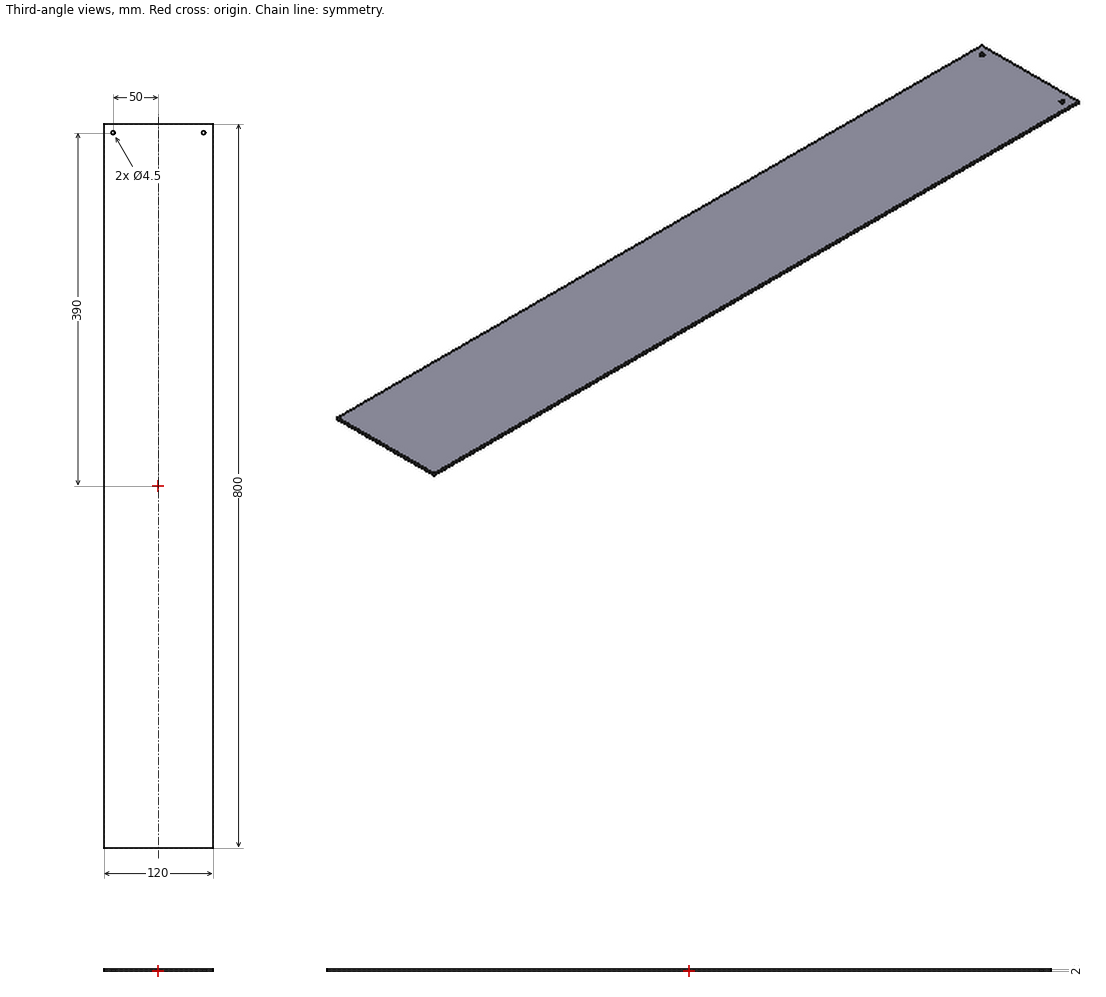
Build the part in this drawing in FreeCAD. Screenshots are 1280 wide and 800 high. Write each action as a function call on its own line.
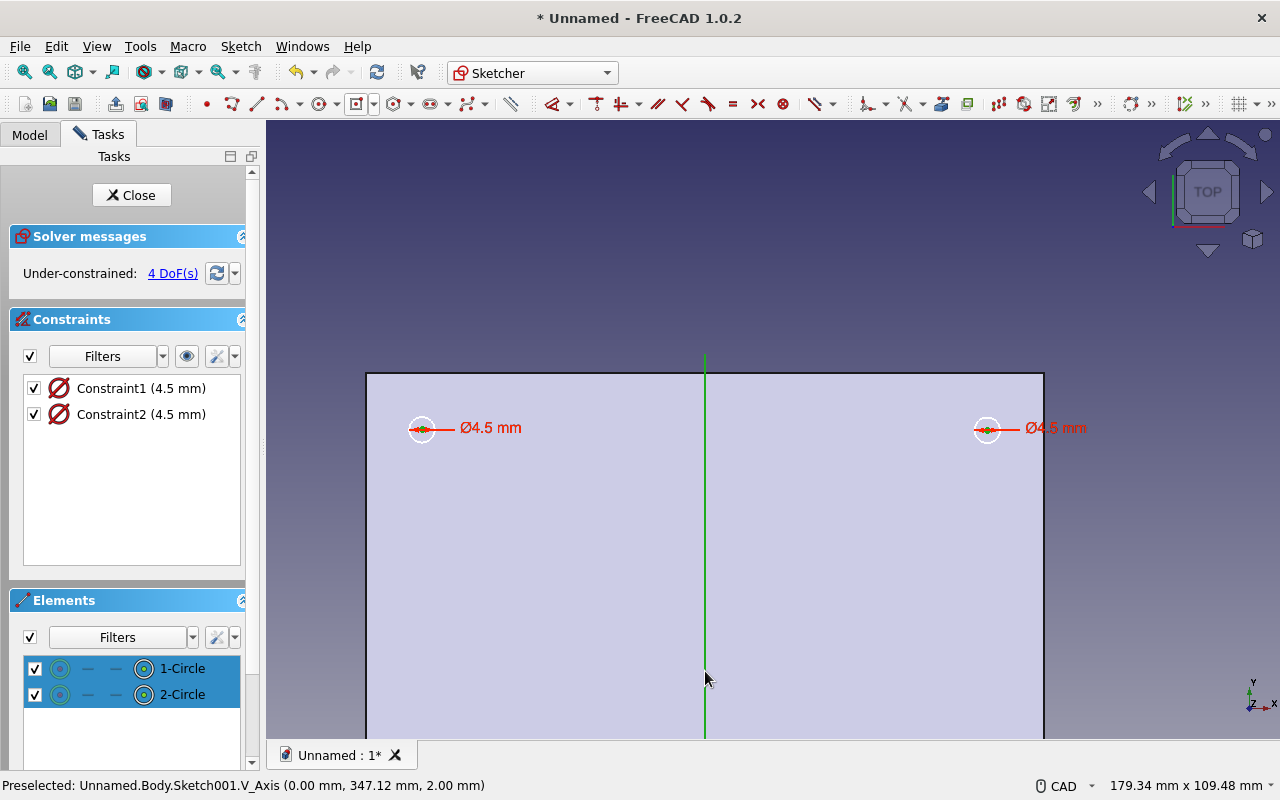
key(s)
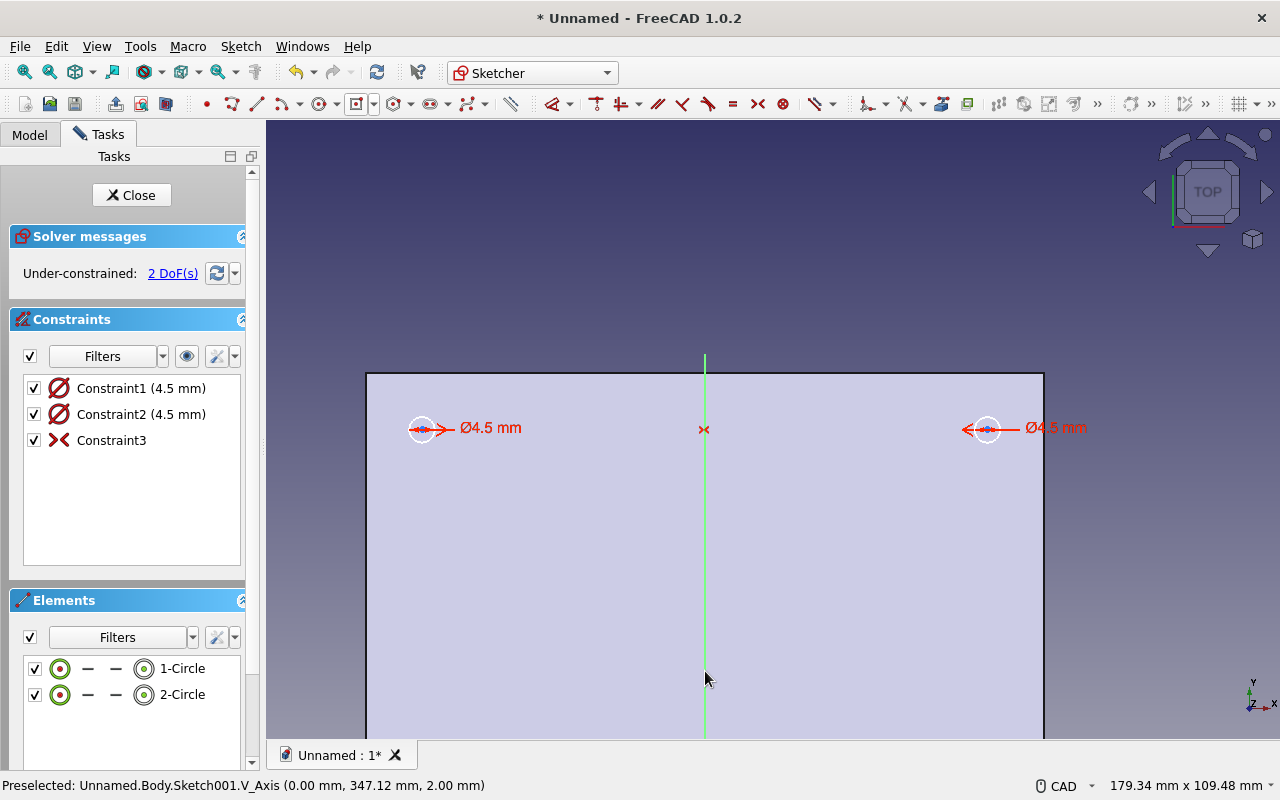
click(552, 104)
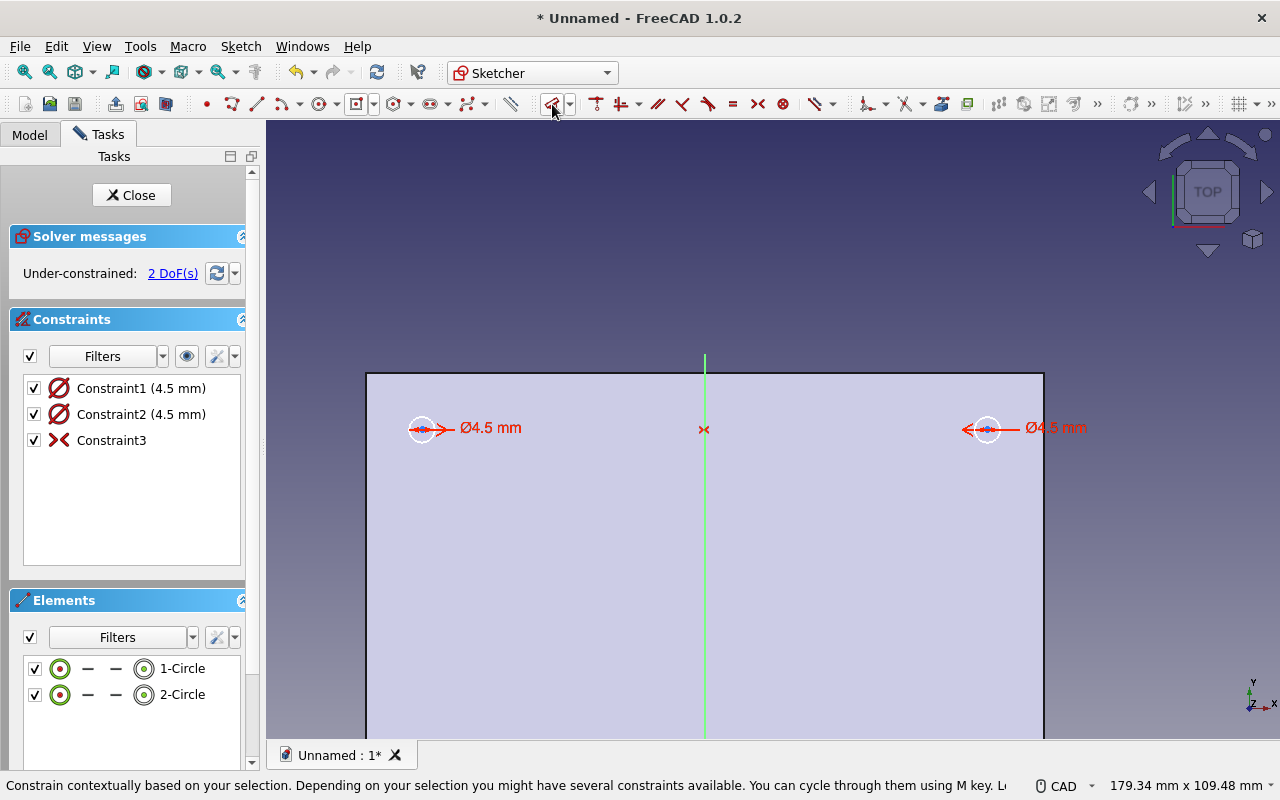
click(422, 430)
click(563, 396)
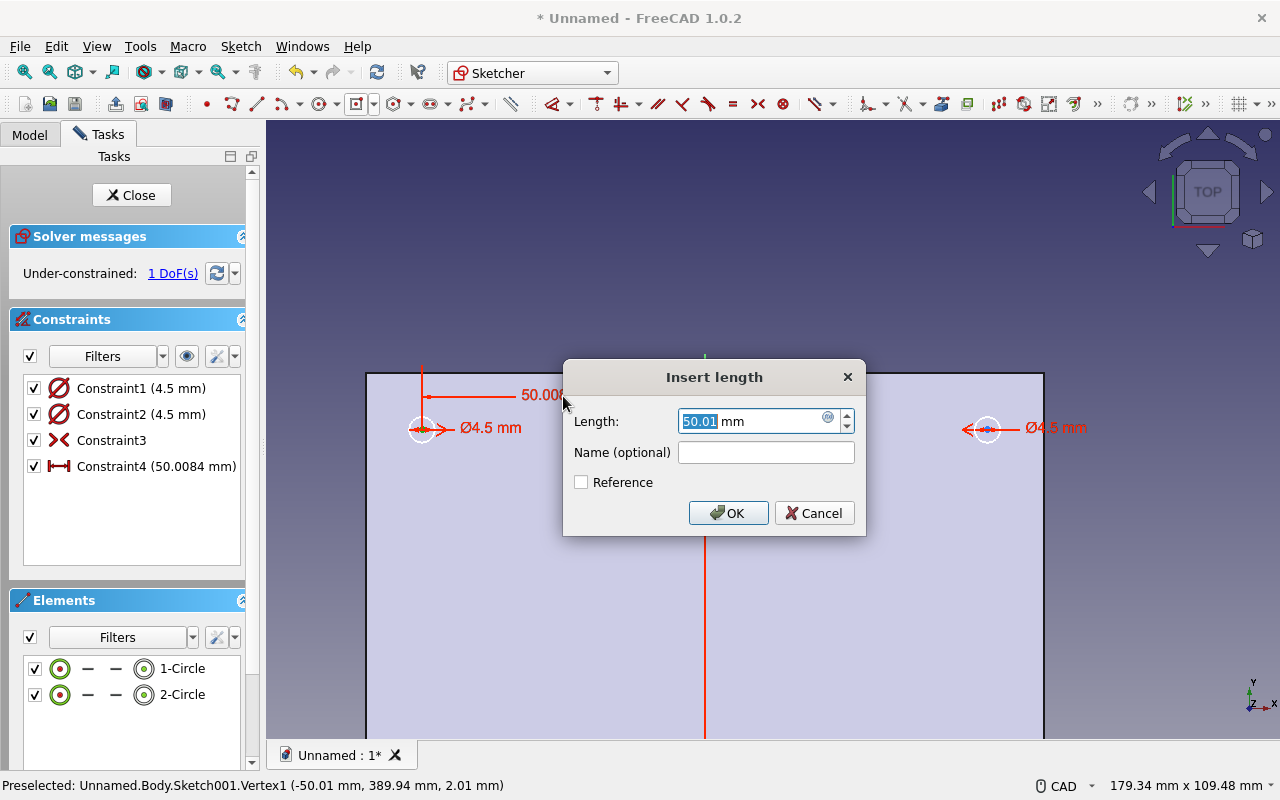
text(50)
key(Return)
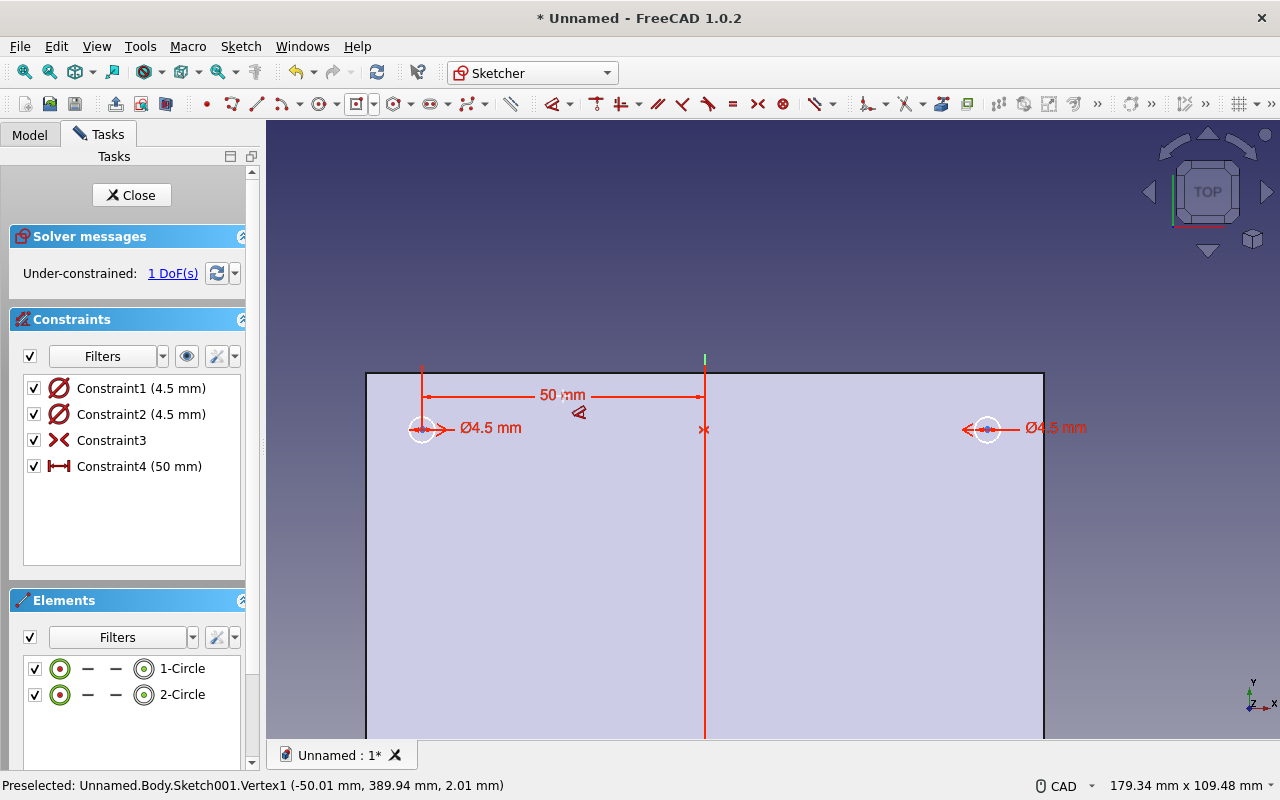
click(422, 430)
click(388, 570)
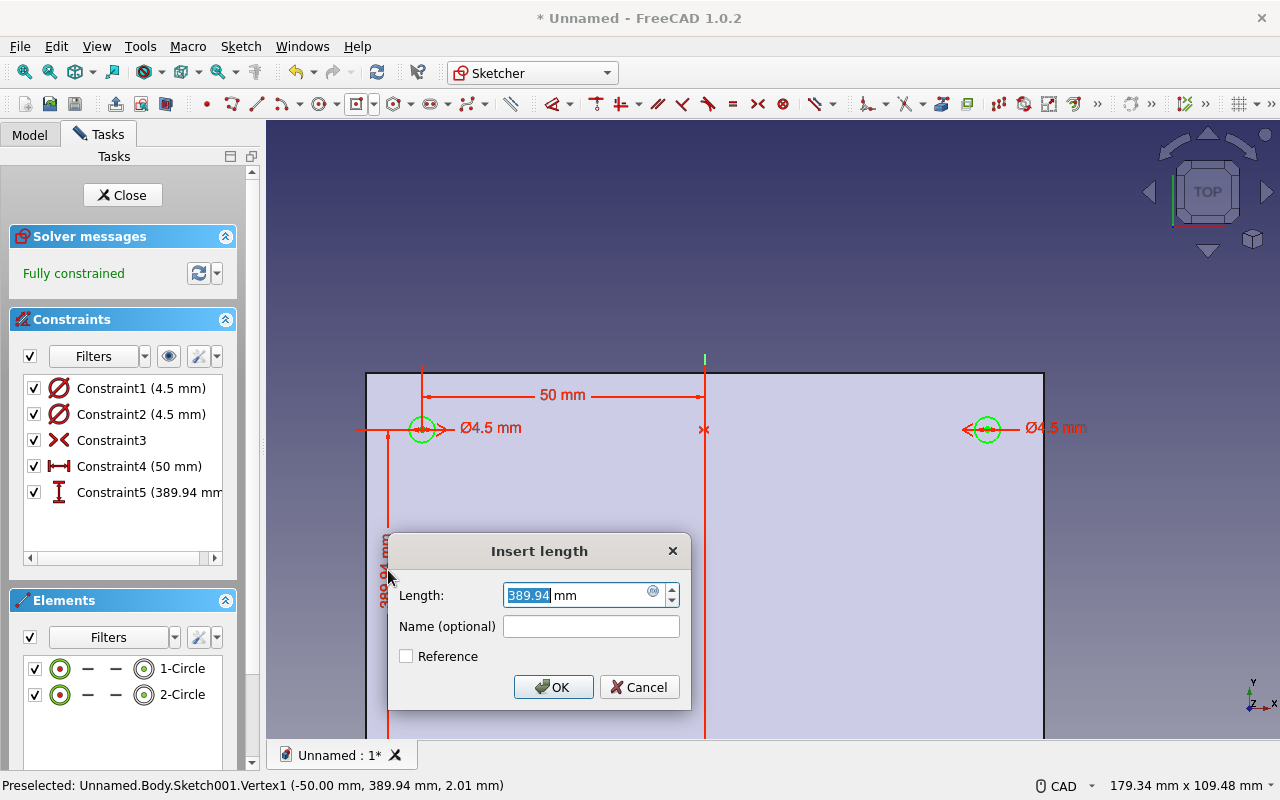
text(390)
key(Return)
key(Escape)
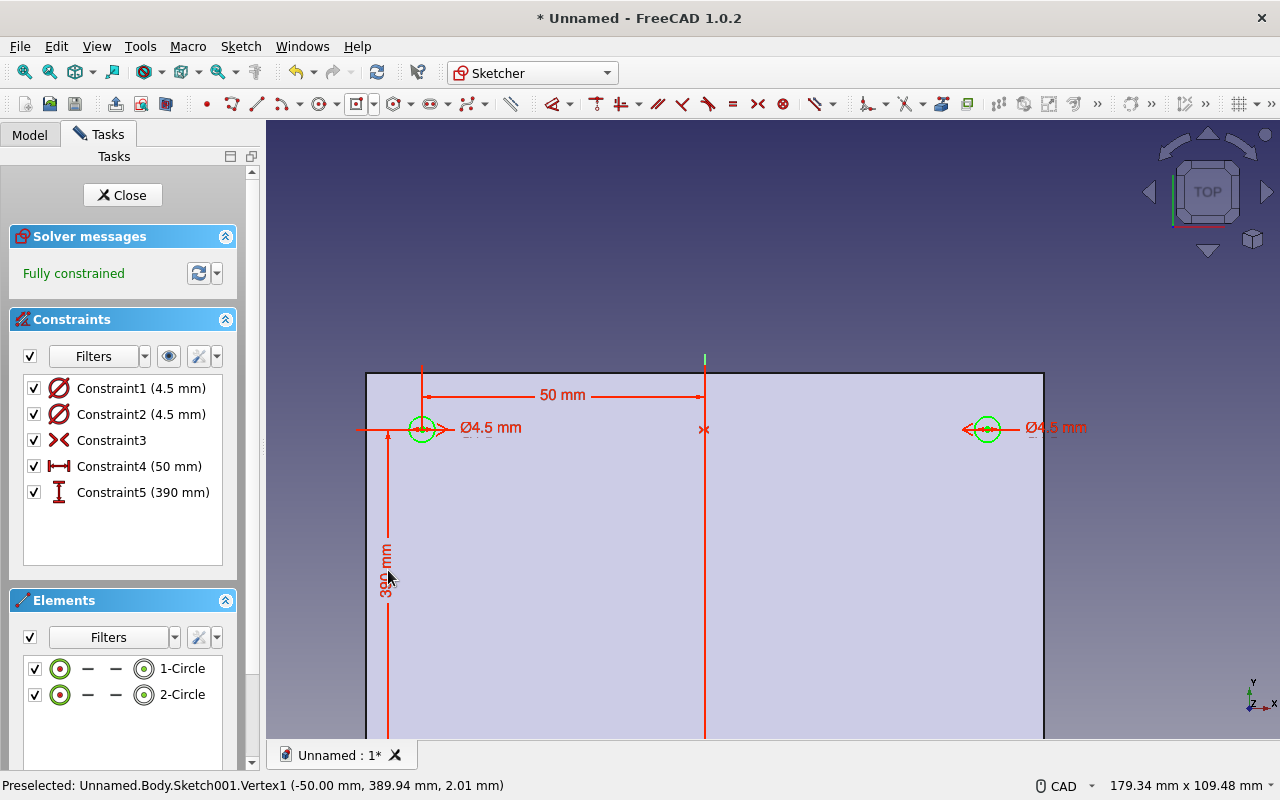
click(123, 195)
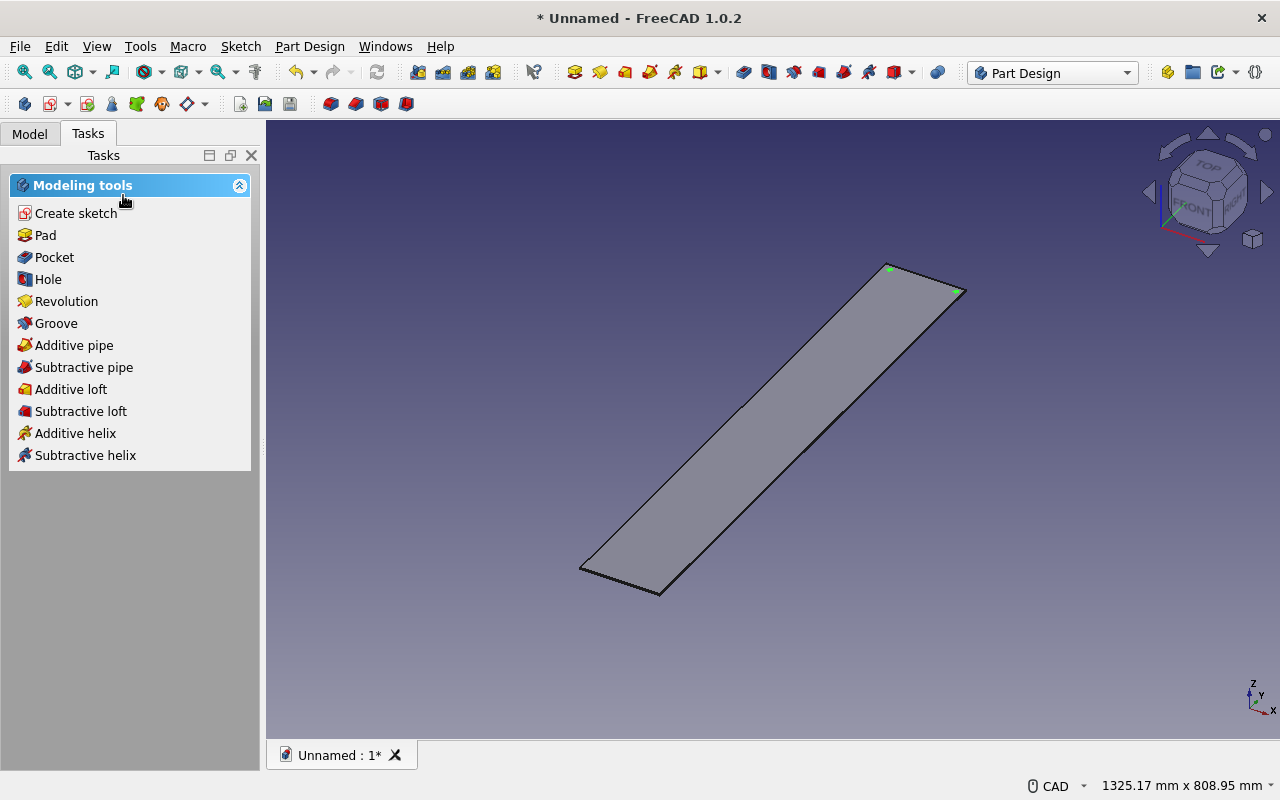
click(744, 72)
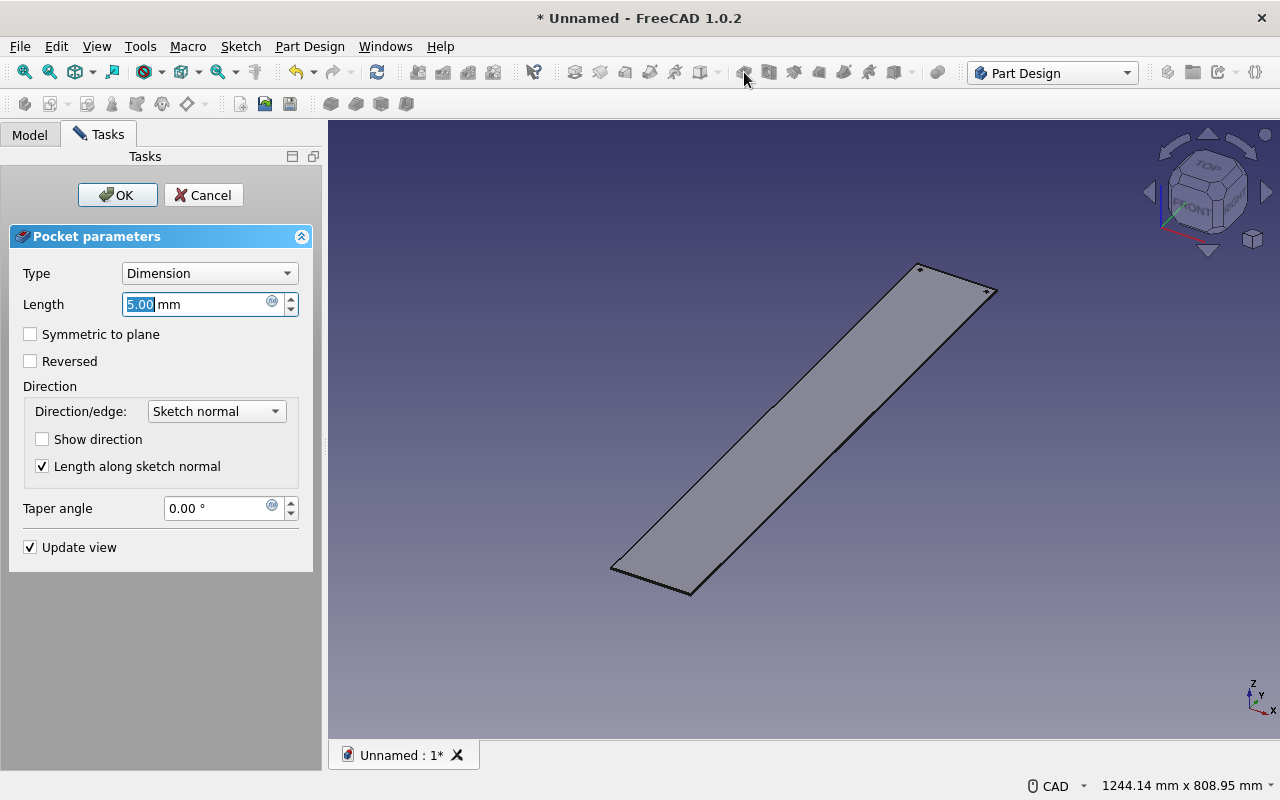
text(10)
key(Tab)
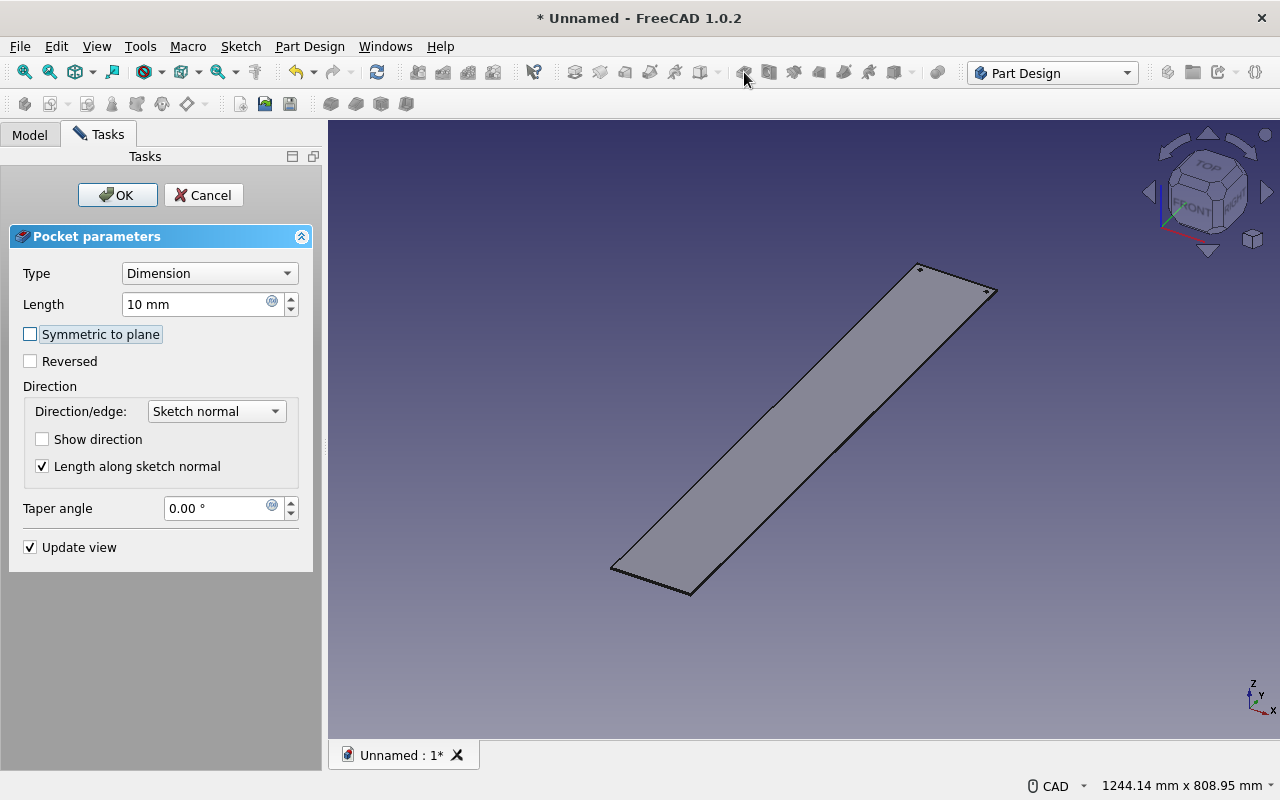
click(118, 195)